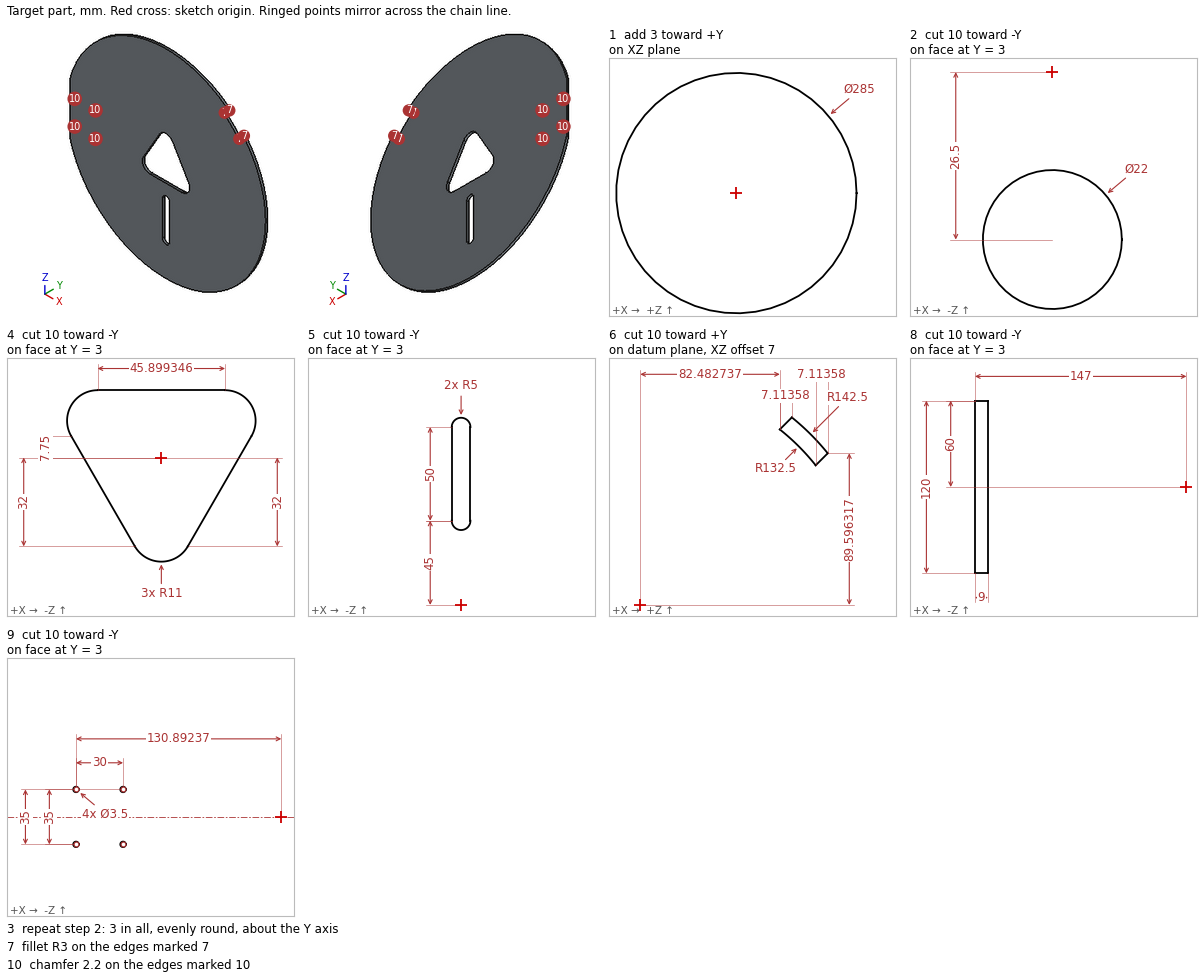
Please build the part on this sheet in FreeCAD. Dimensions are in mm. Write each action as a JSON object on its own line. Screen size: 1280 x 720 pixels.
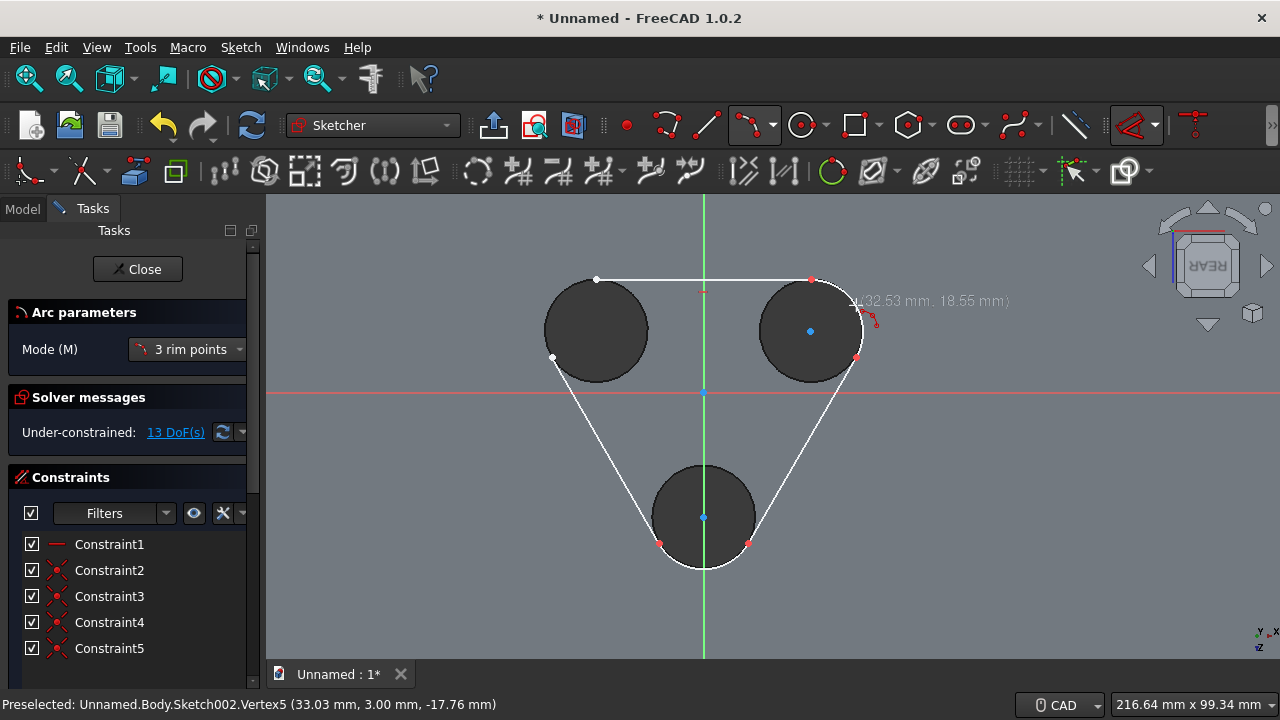
{"action": "left_click", "coordinate": [596, 280]}
{"action": "left_click", "coordinate": [552, 358]}
{"action": "left_click", "coordinate": [552, 305]}
{"action": "key", "text": "Escape"}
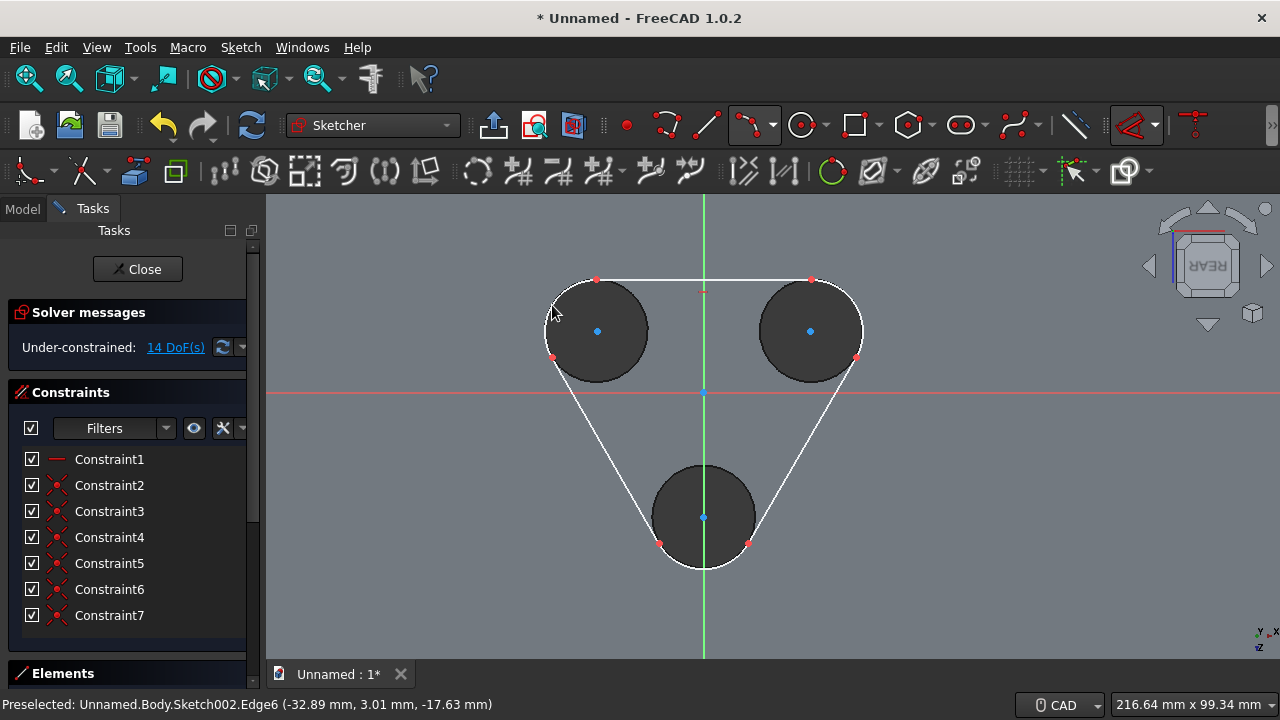
{"action": "left_click", "coordinate": [584, 414]}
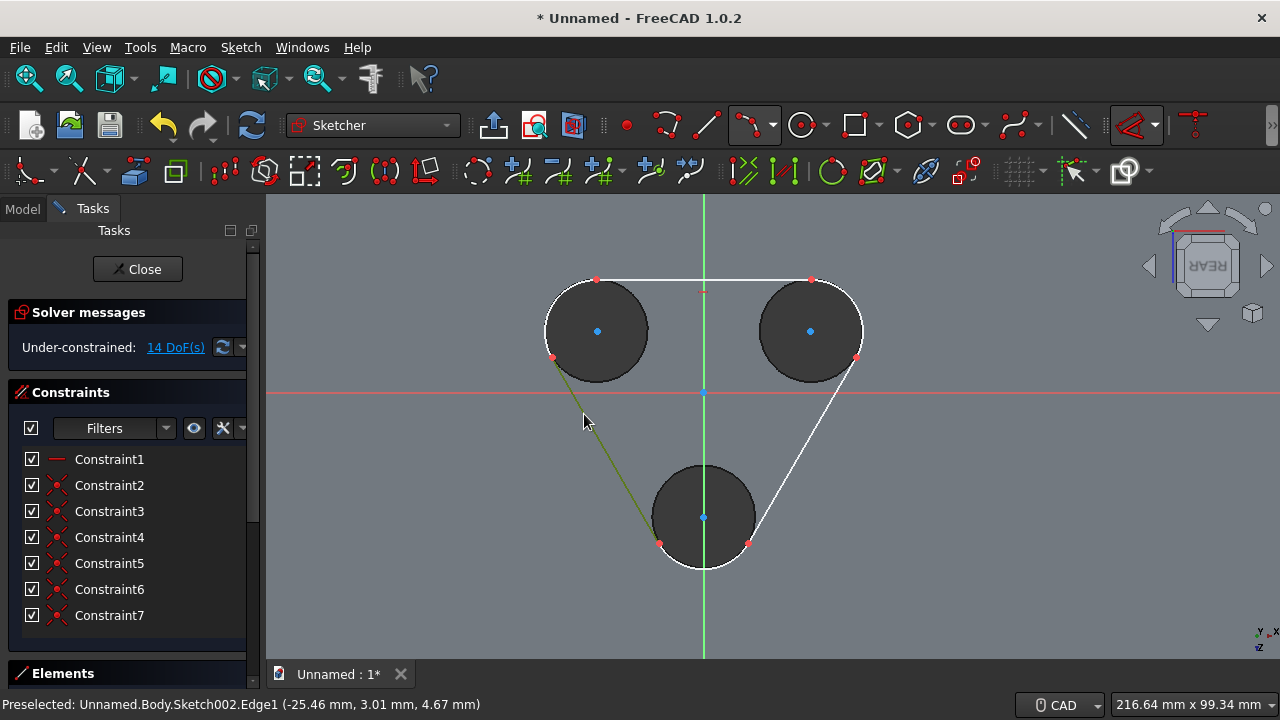
{"action": "left_click", "coordinate": [683, 565]}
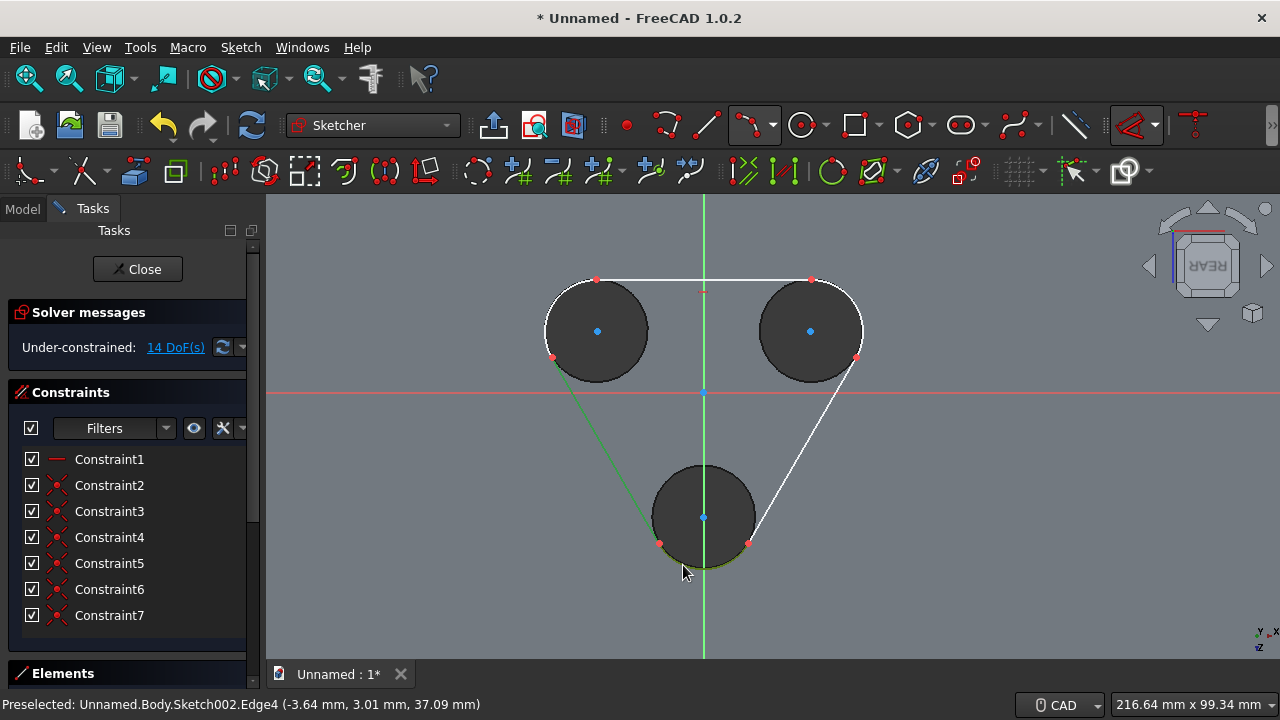
{"action": "key", "text": "t"}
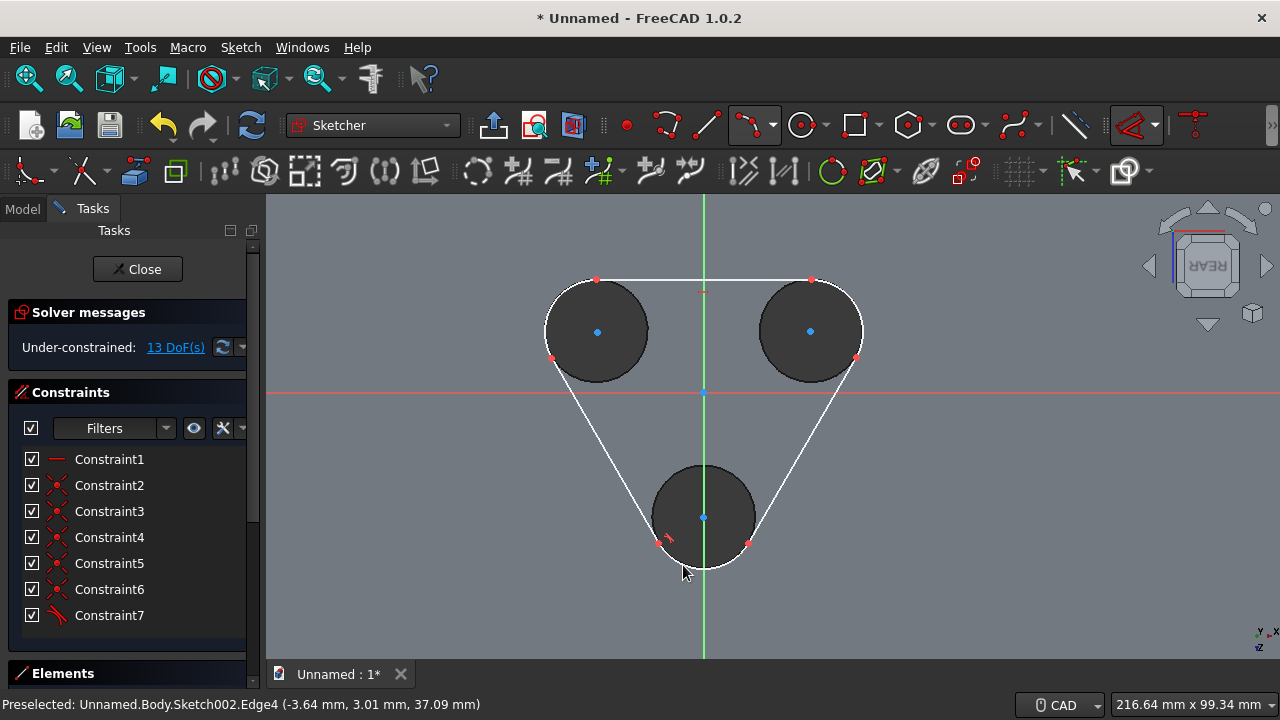
{"action": "left_click", "coordinate": [584, 414]}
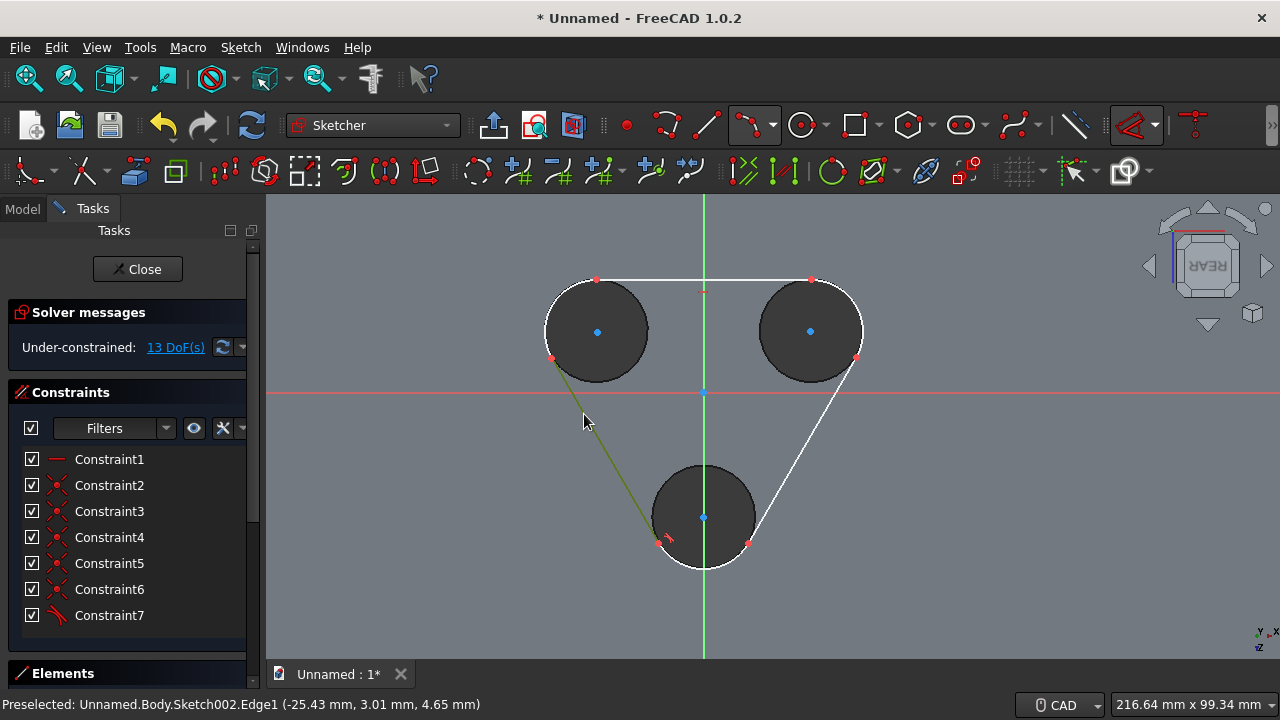
{"action": "left_click", "coordinate": [566, 290]}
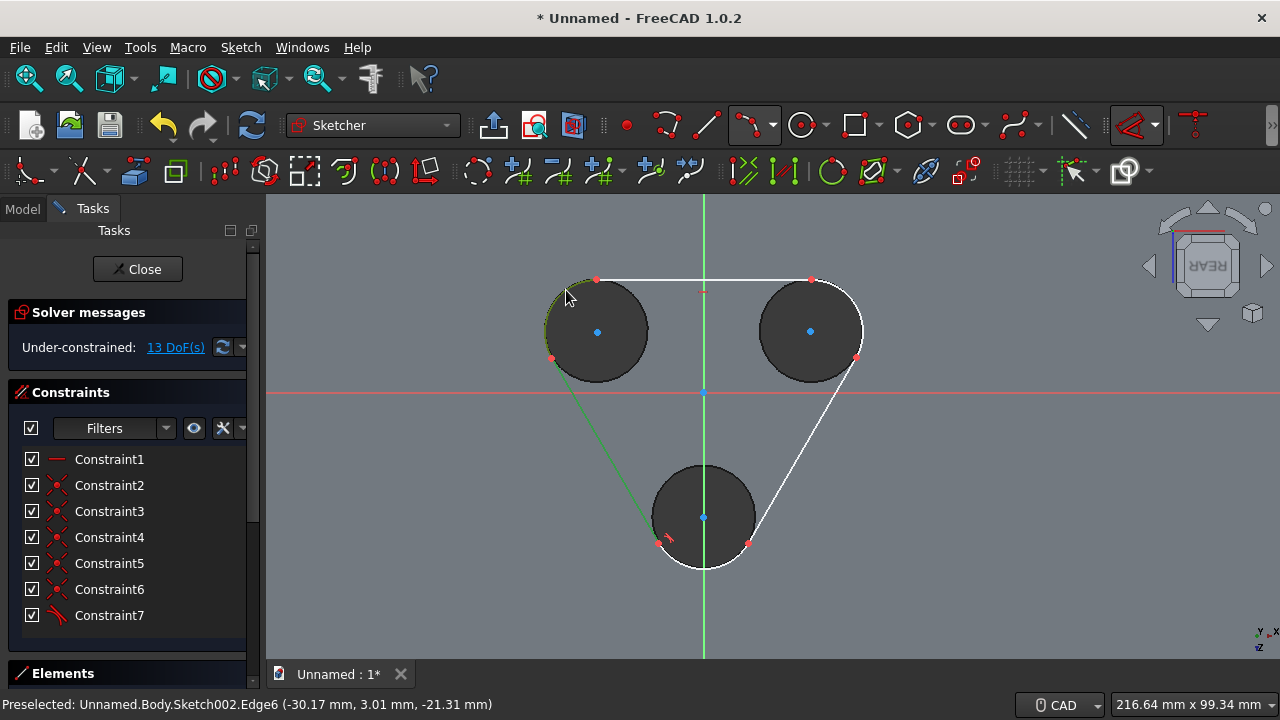
{"action": "key", "text": "t"}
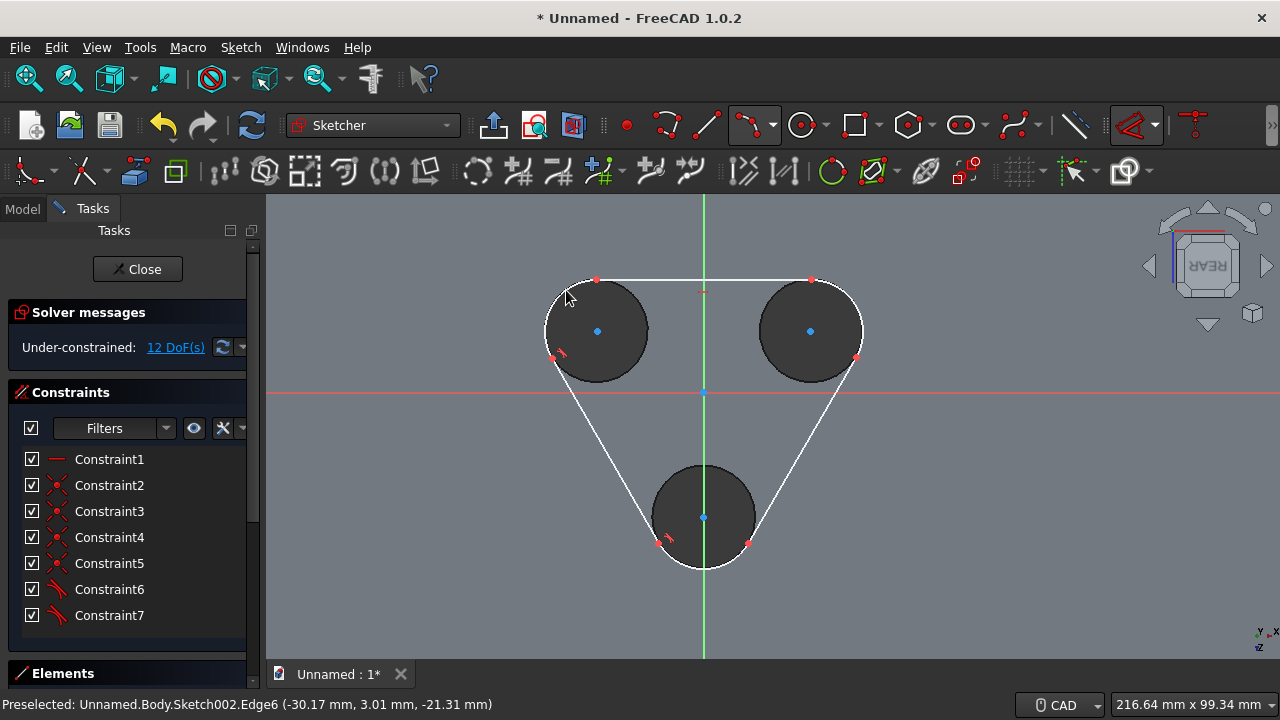
{"action": "left_click", "coordinate": [780, 488]}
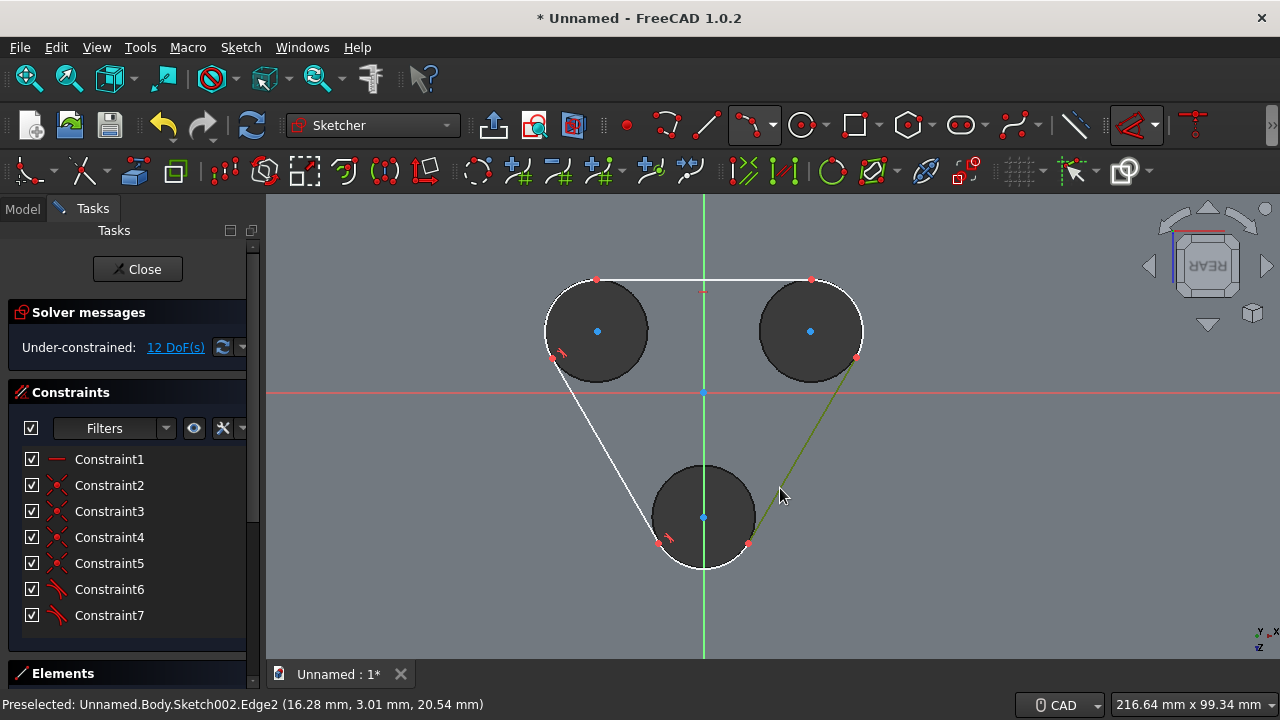
{"action": "left_click", "coordinate": [682, 564]}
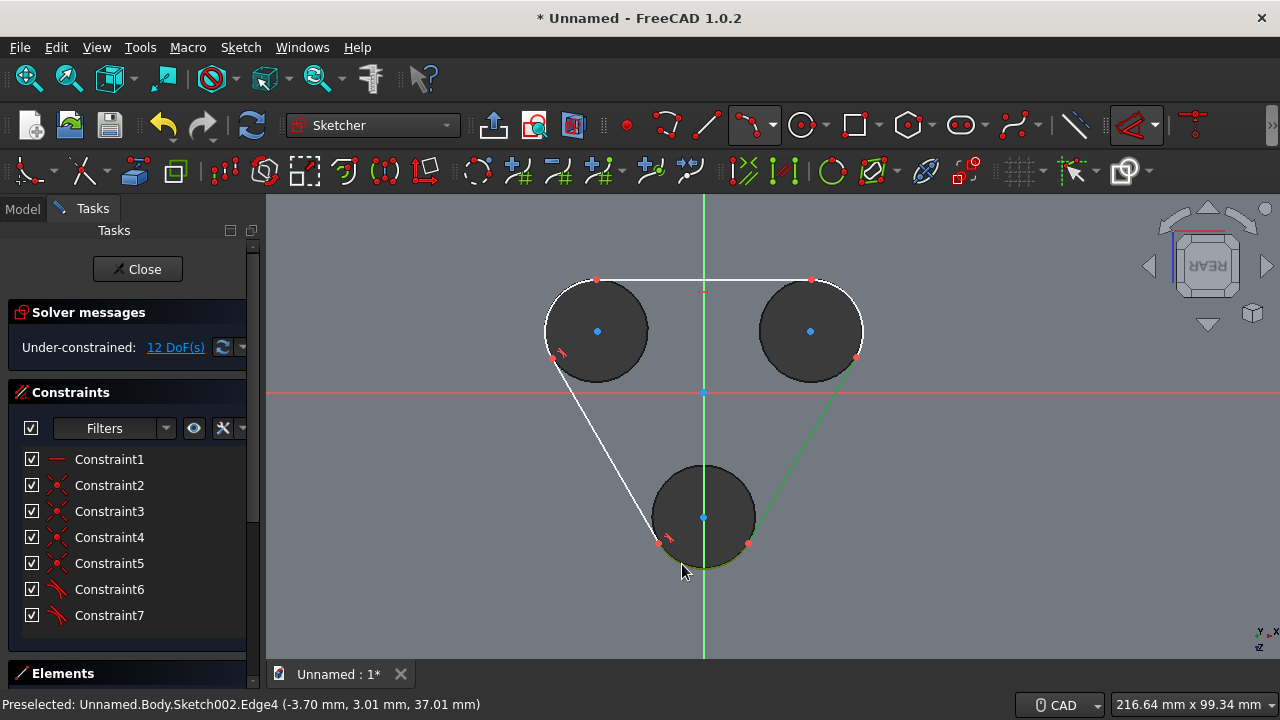
{"action": "key", "text": "t"}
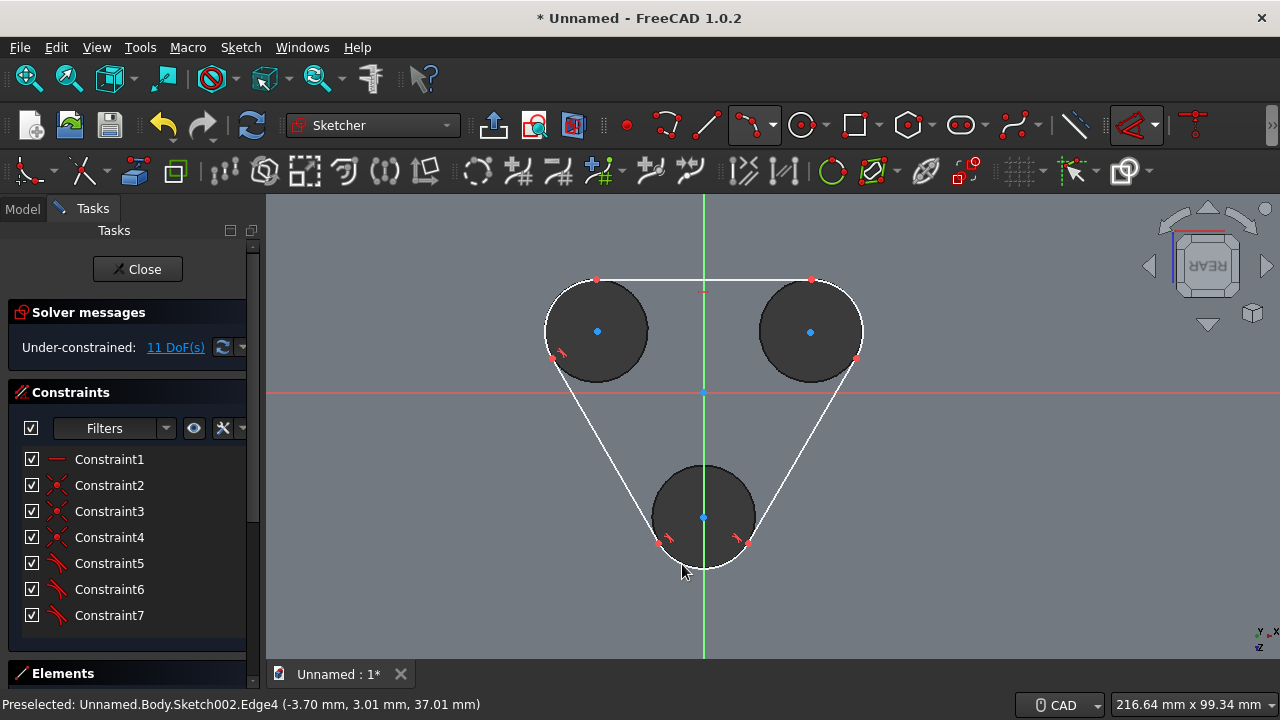
{"action": "left_click", "coordinate": [780, 488]}